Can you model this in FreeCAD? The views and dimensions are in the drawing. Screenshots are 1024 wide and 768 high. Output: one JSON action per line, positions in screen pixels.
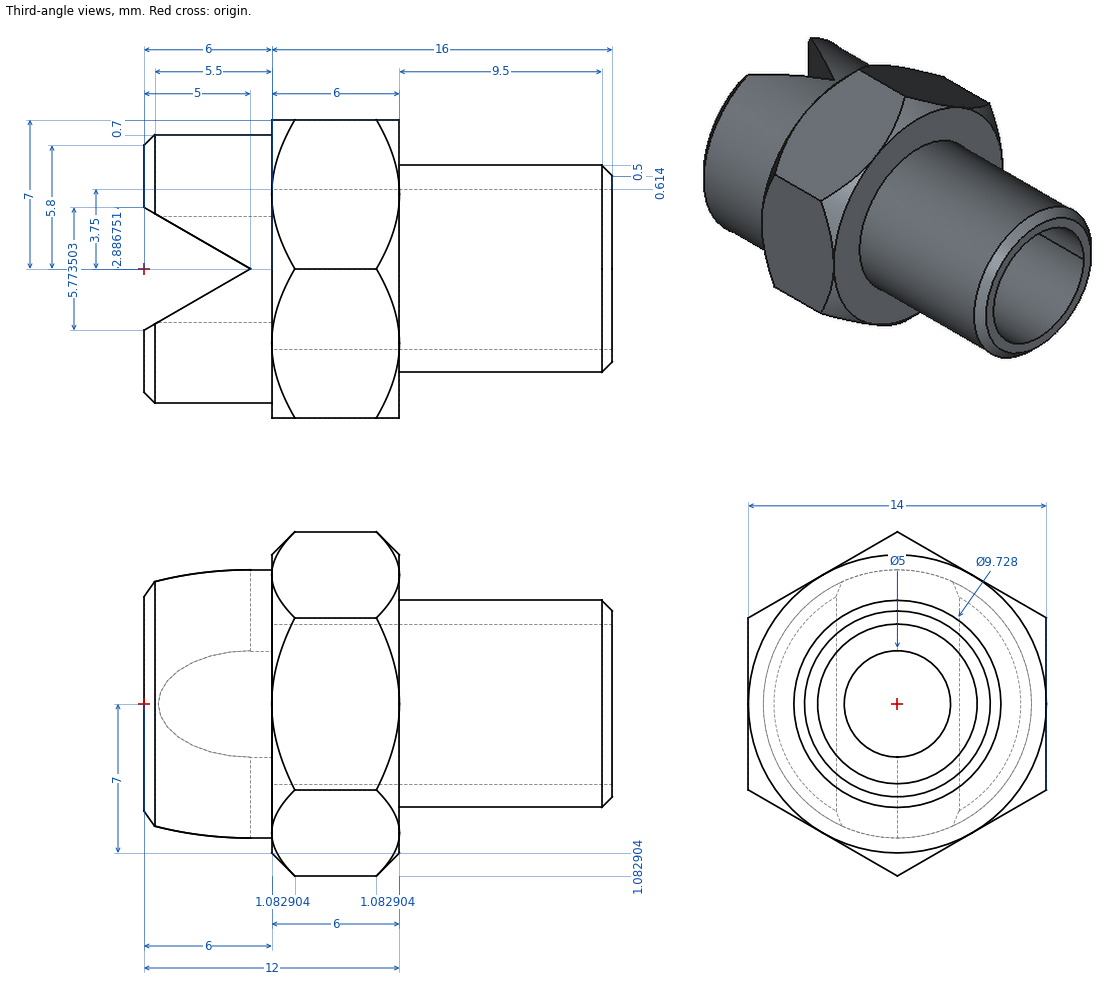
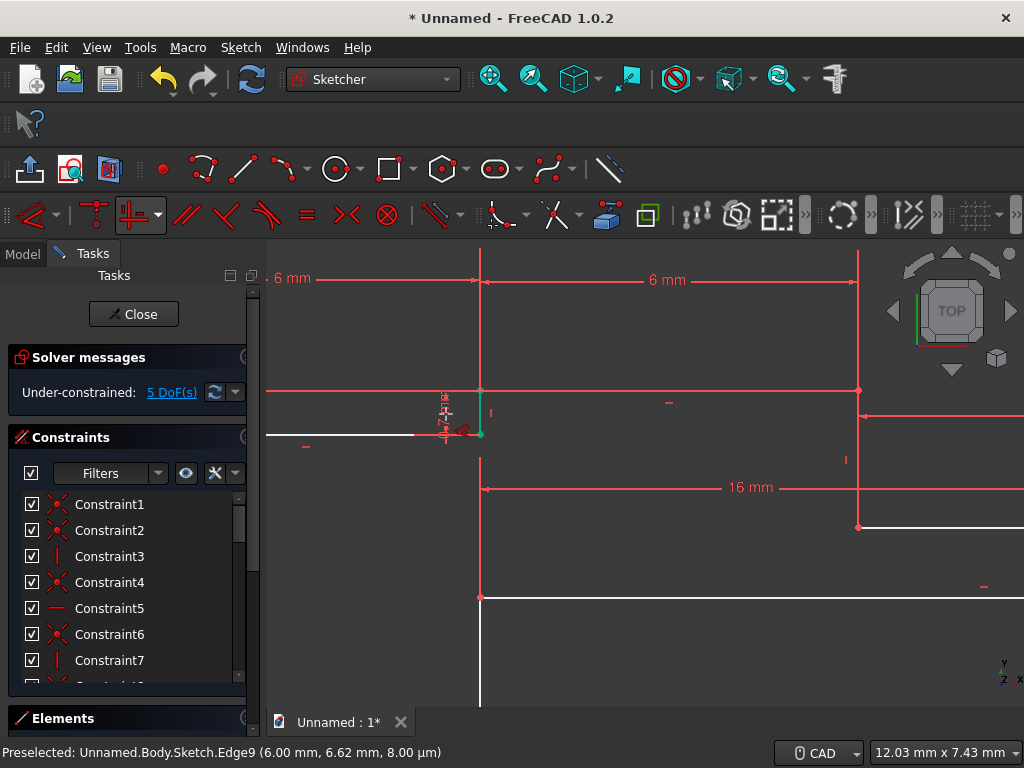
{"action": "left_click", "coordinate": [376, 435]}
{"action": "left_click", "coordinate": [344, 401]}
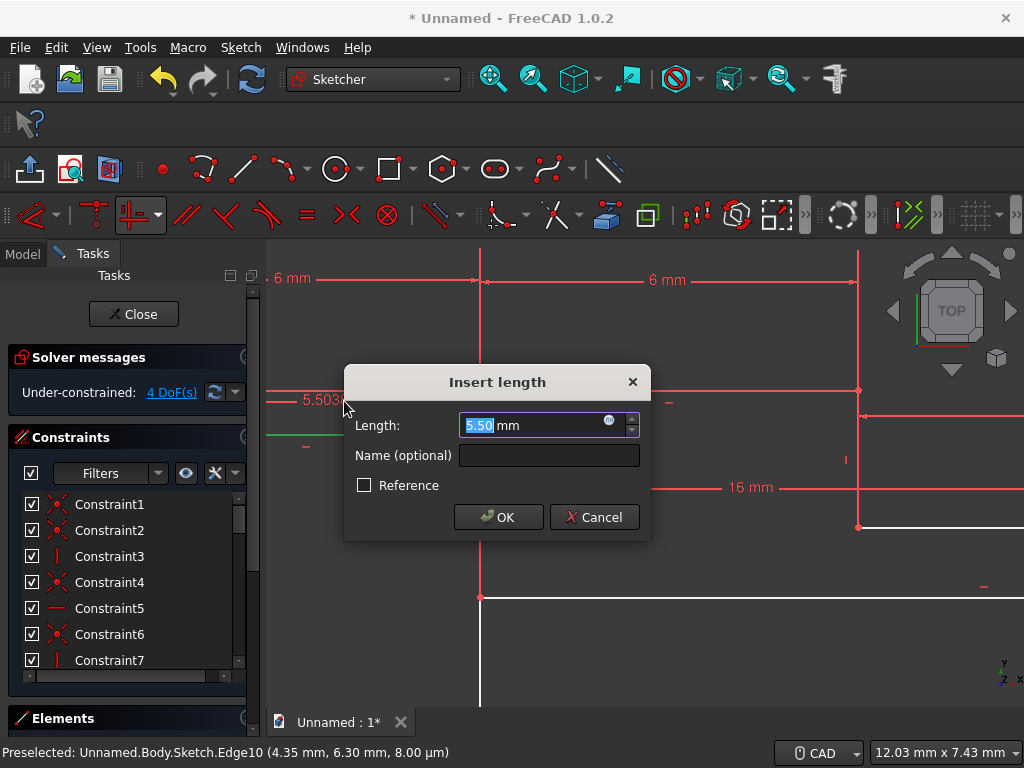
{"action": "type", "text": "5.5"}
{"action": "key", "text": "Return"}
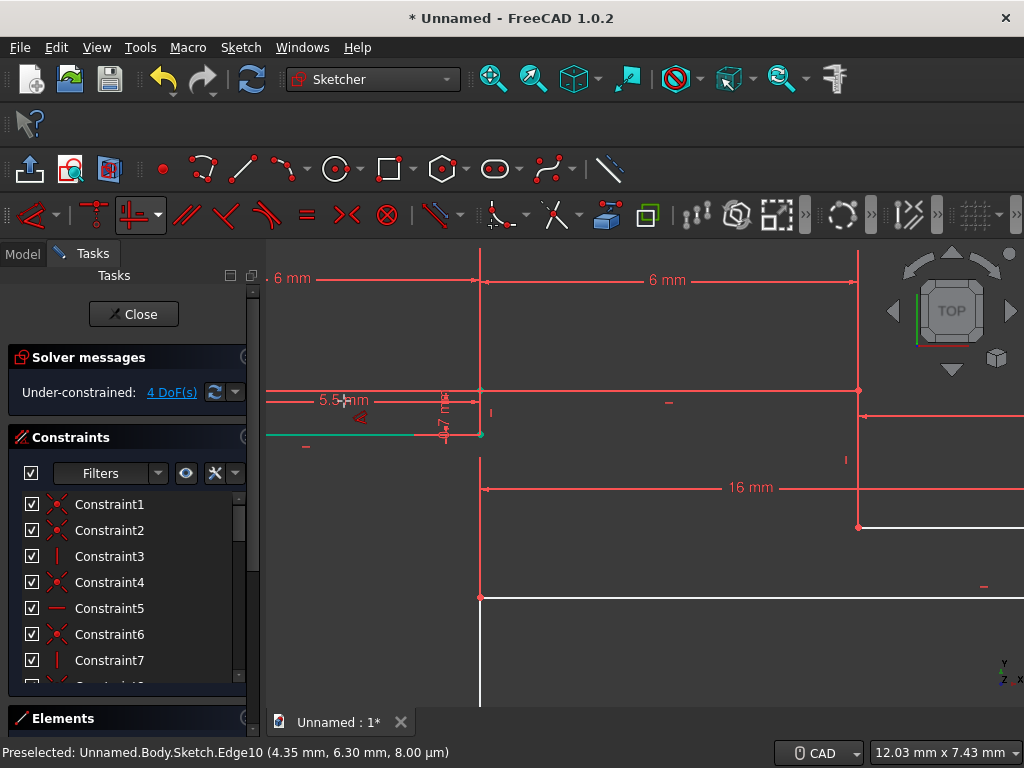
{"action": "scroll", "coordinate": [482, 413], "scroll_direction": "down", "scroll_amount": 6}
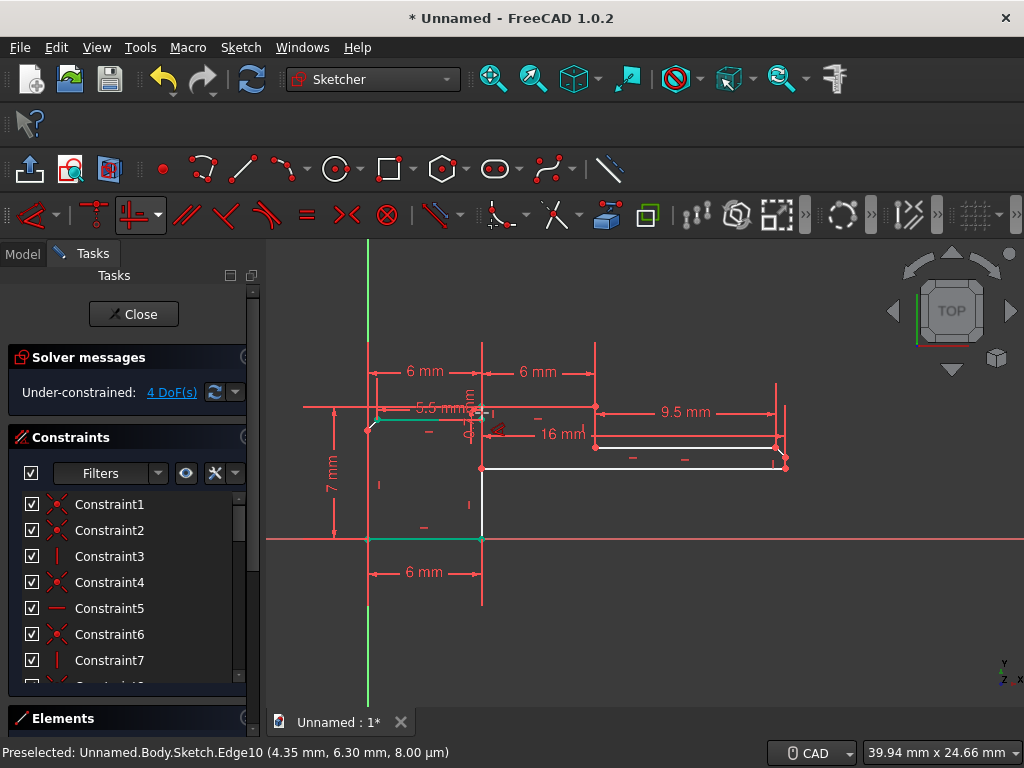
{"action": "left_click", "coordinate": [368, 463]}
{"action": "left_click", "coordinate": [334, 510]}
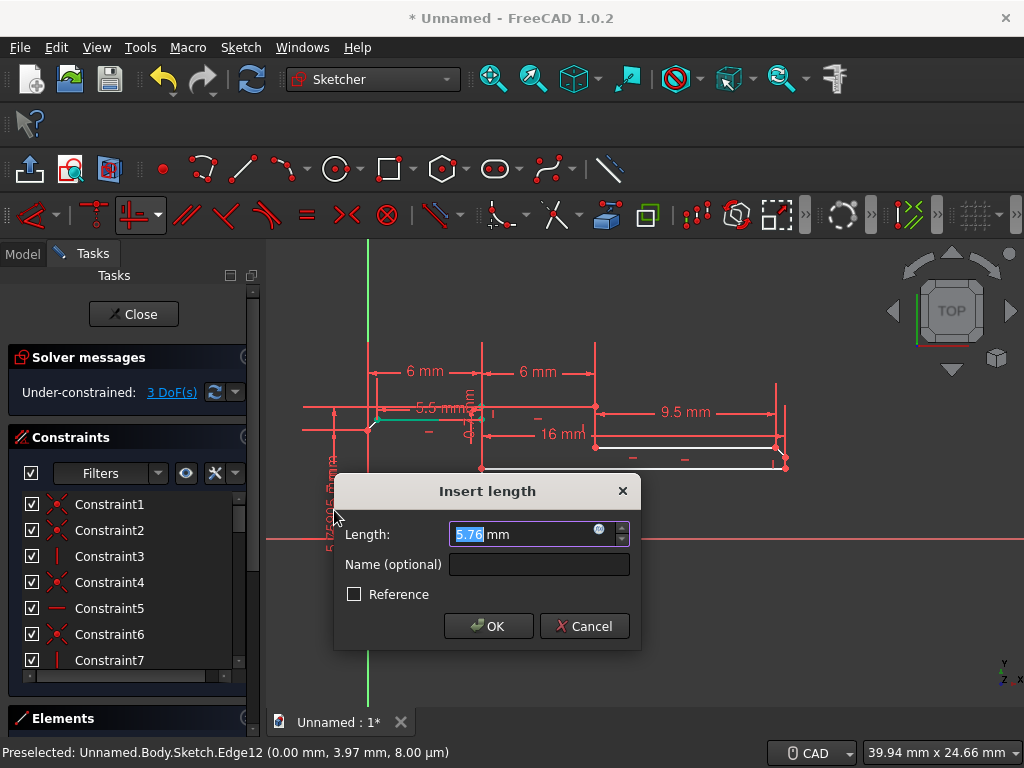
{"action": "type", "text": "5.8"}
{"action": "key", "text": "Return"}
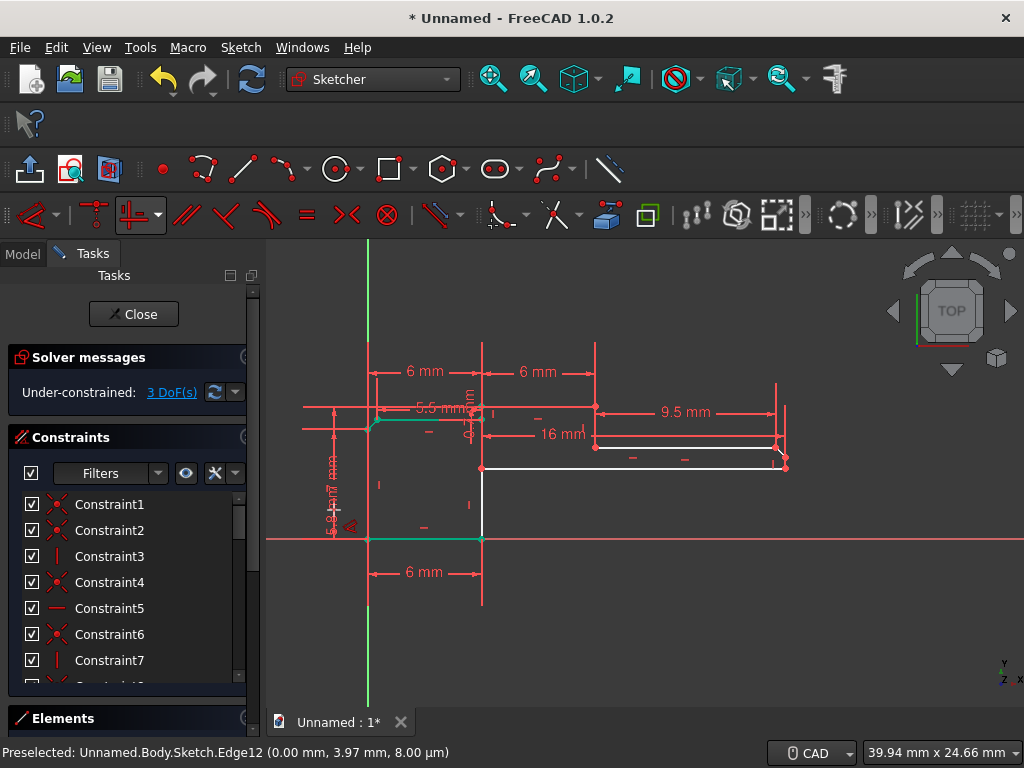
{"action": "left_click", "coordinate": [482, 518]}
{"action": "left_click", "coordinate": [448, 504]}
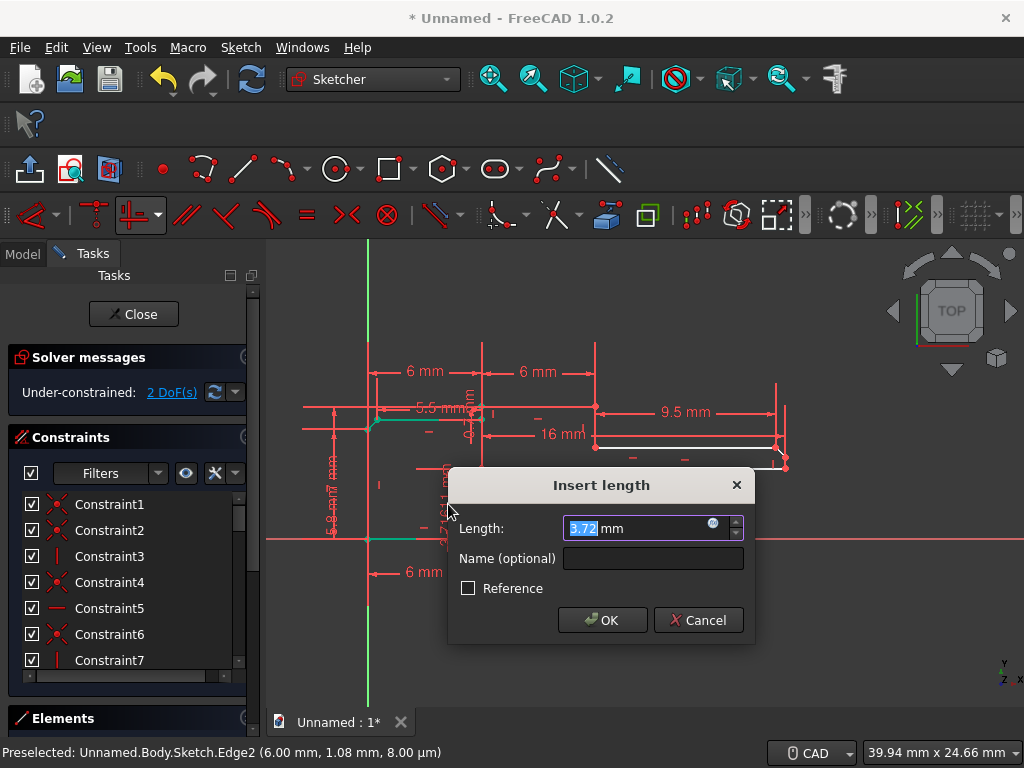
{"action": "type", "text": "3.75"}
{"action": "key", "text": "Return"}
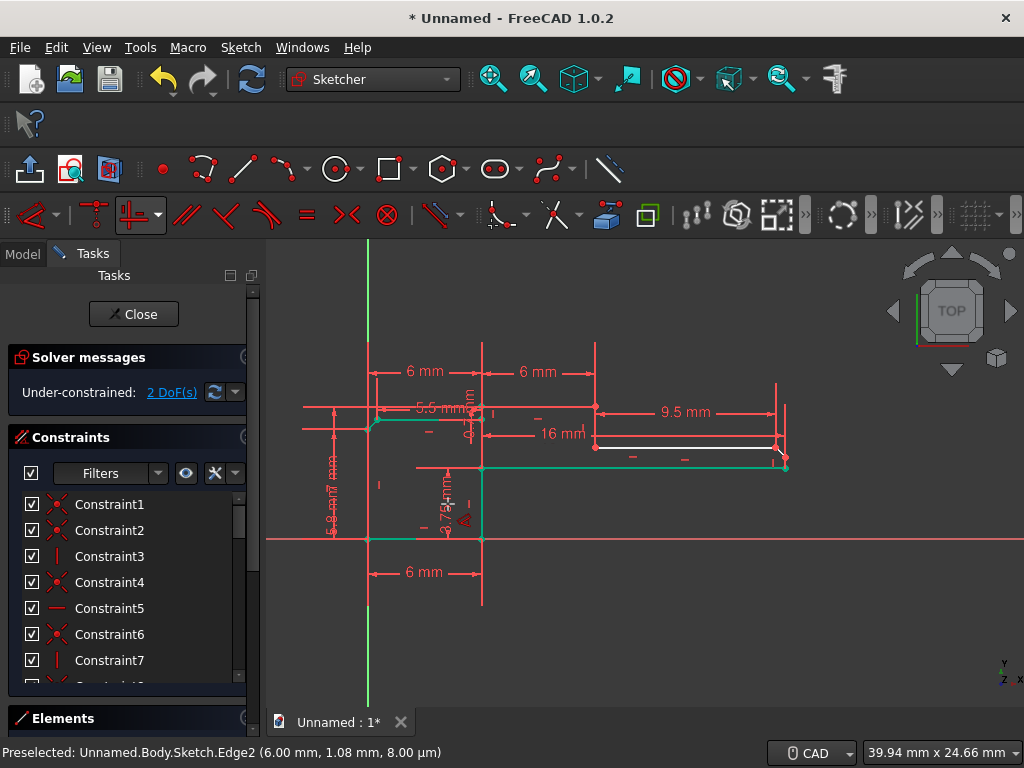
{"action": "scroll", "coordinate": [781, 452], "scroll_direction": "up", "scroll_amount": 8}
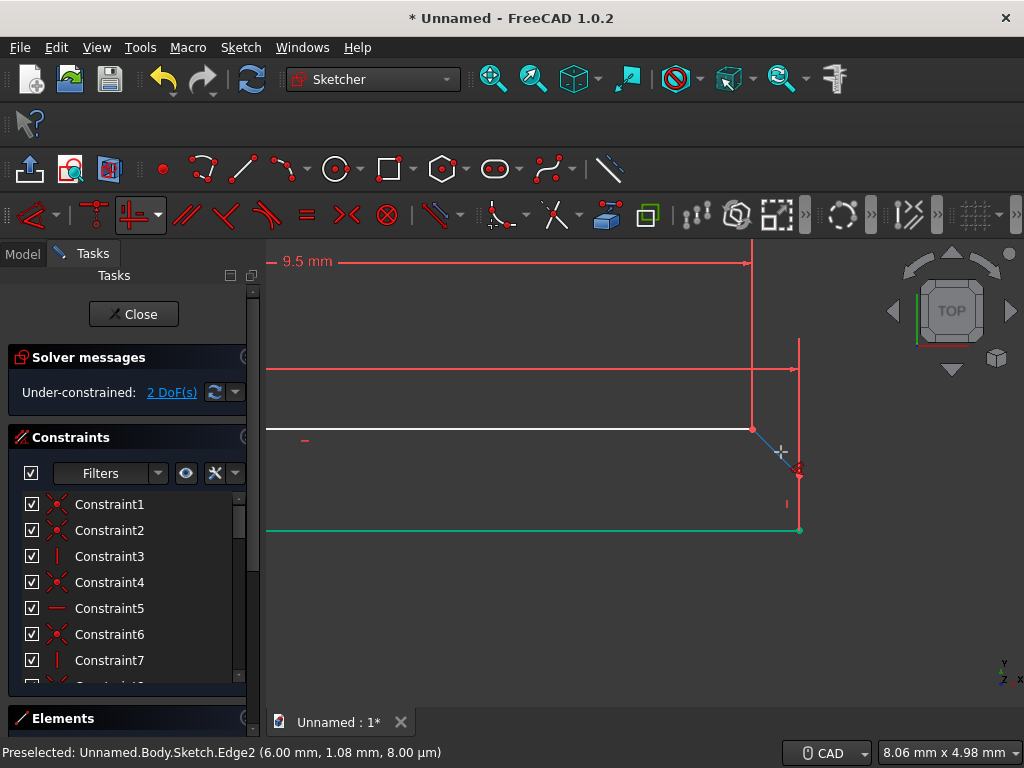
{"action": "left_click", "coordinate": [776, 452]}
{"action": "left_click", "coordinate": [833, 452]}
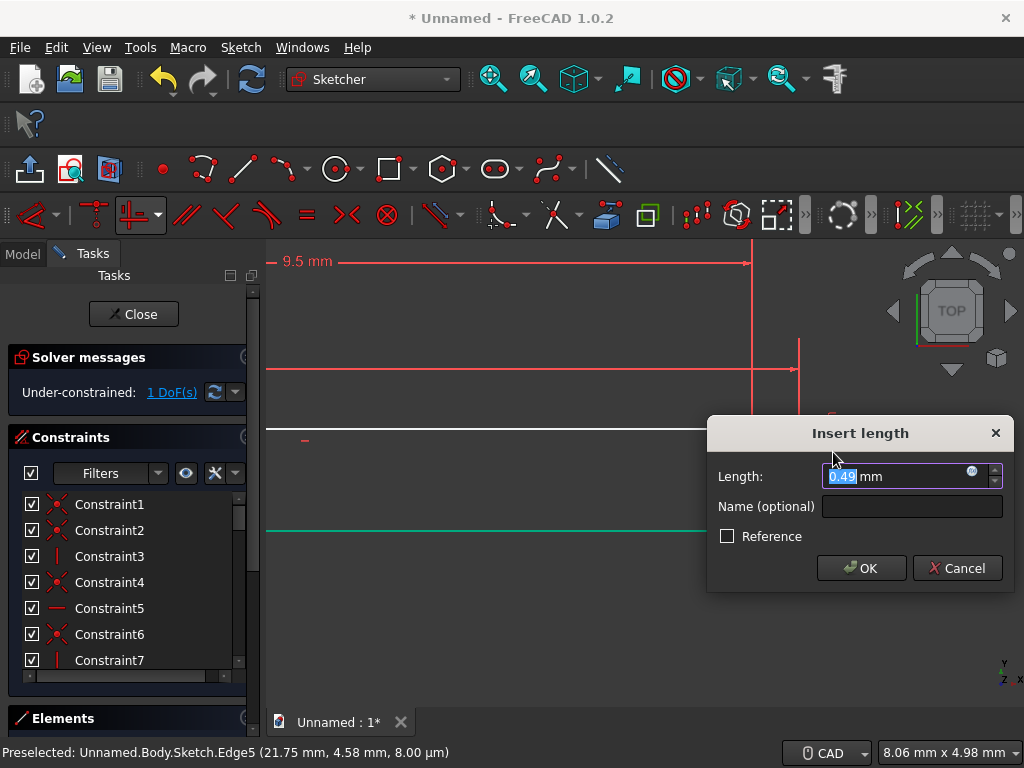
{"action": "type", "text": "0.5"}
{"action": "key", "text": "Return"}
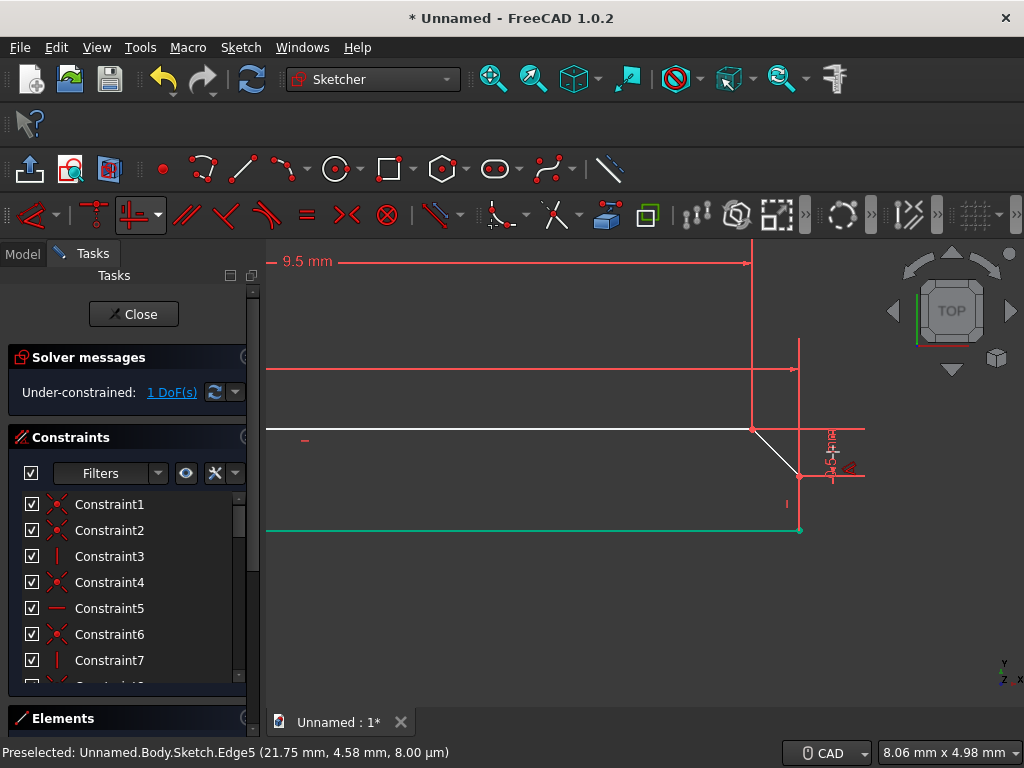
{"action": "left_click", "coordinate": [799, 514]}
{"action": "left_click", "coordinate": [833, 503]}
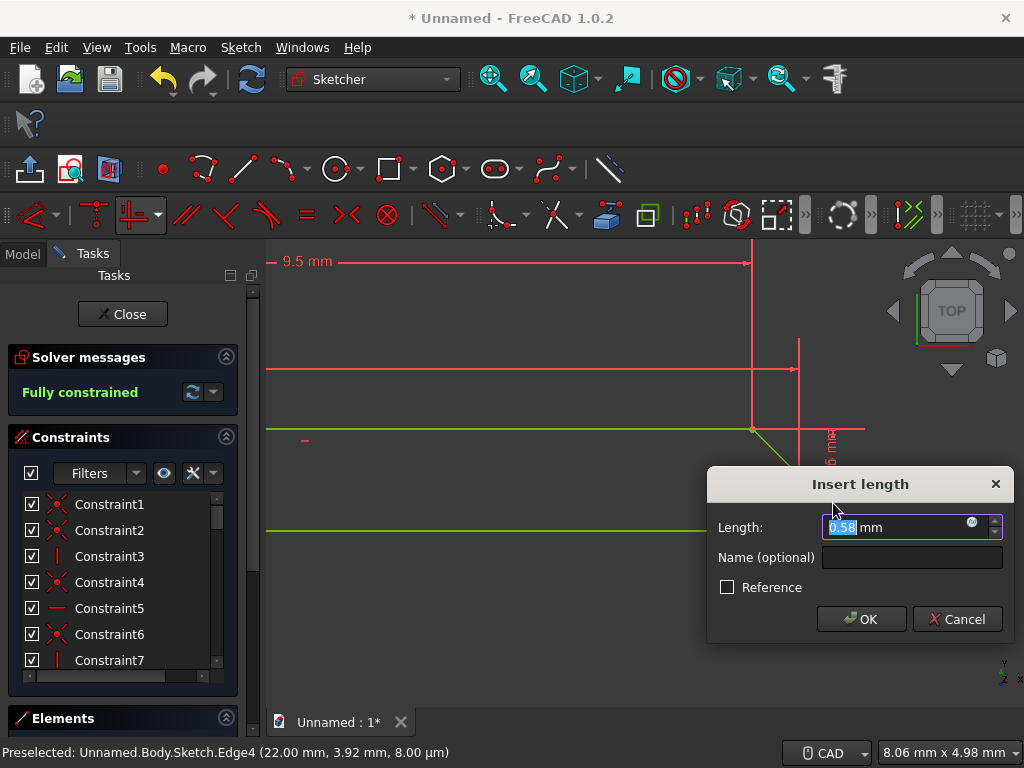
{"action": "type", "text": "0.614"}
{"action": "key", "text": "Return"}
{"action": "key", "text": "Escape"}